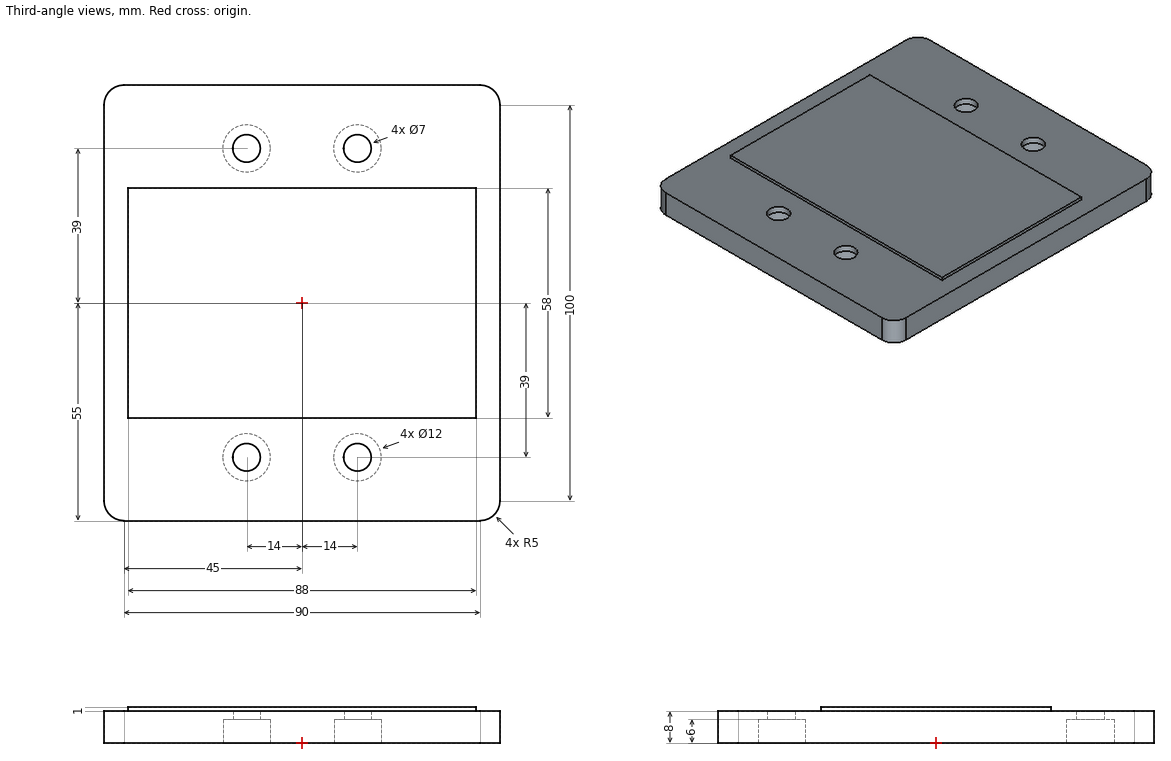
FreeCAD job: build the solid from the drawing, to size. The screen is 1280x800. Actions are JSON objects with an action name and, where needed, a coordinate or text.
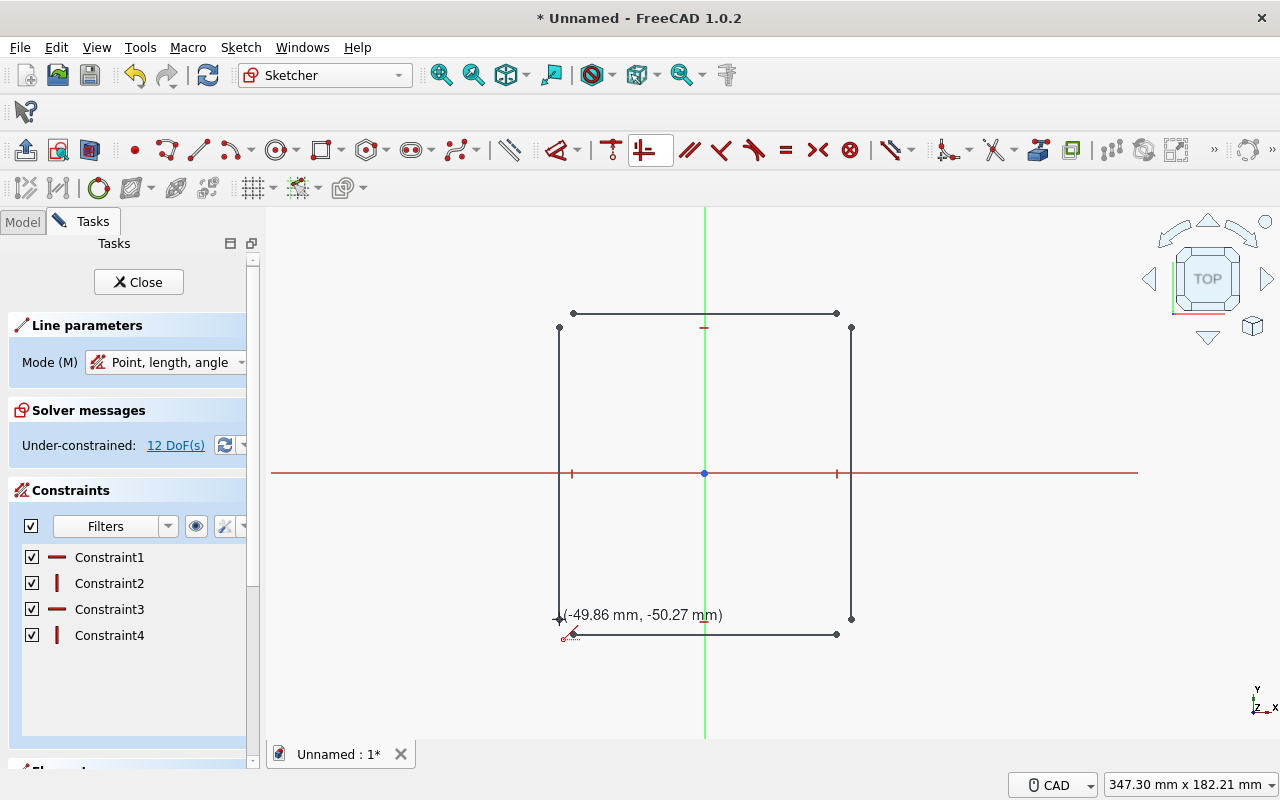
{"action": "left_click", "coordinate": [254, 150]}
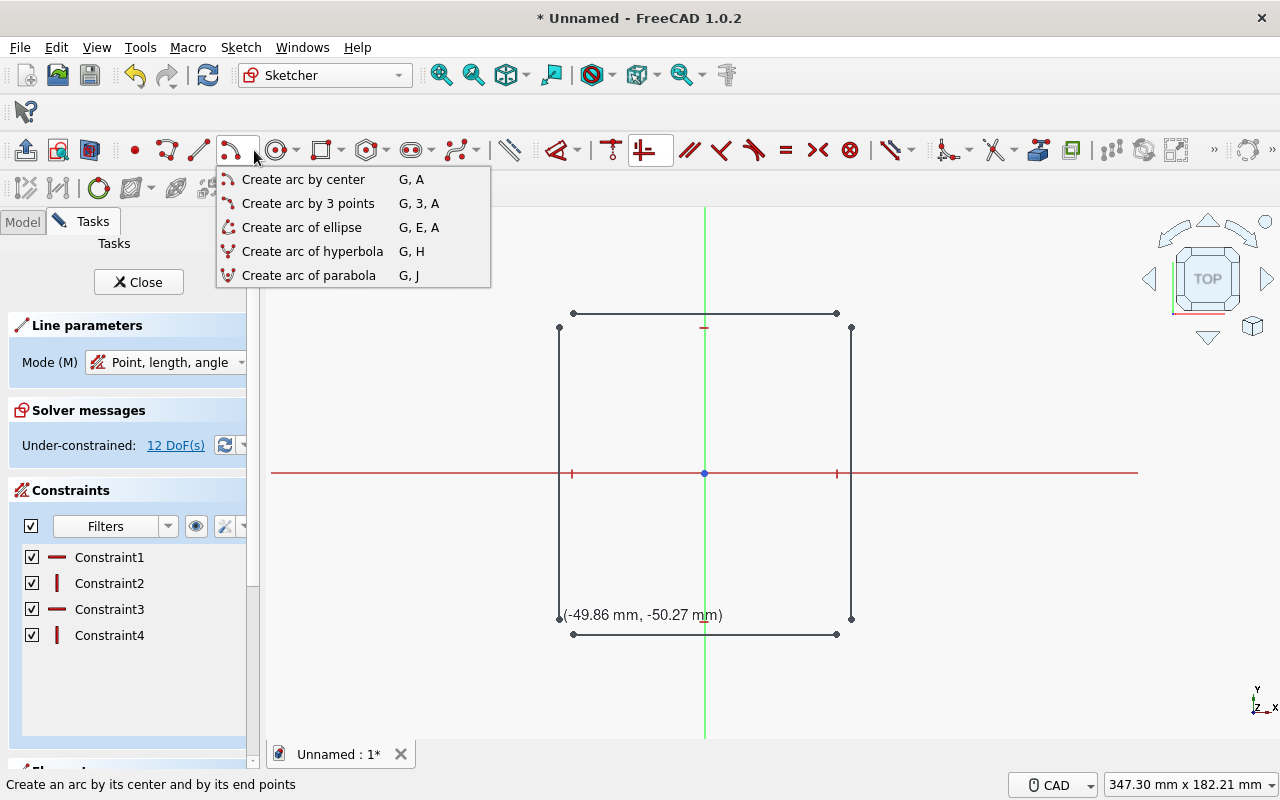
{"action": "left_click", "coordinate": [354, 203]}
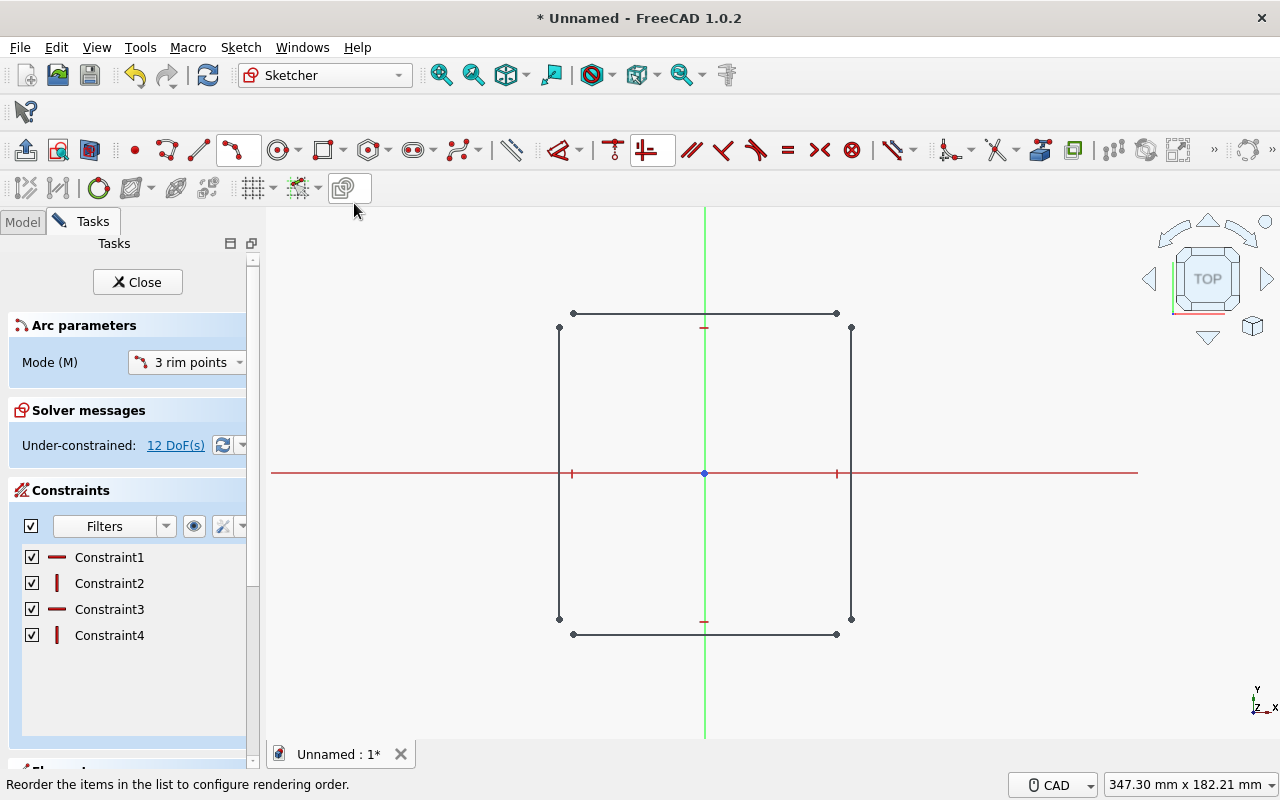
{"action": "left_click", "coordinate": [836, 635]}
{"action": "left_click", "coordinate": [851, 620]}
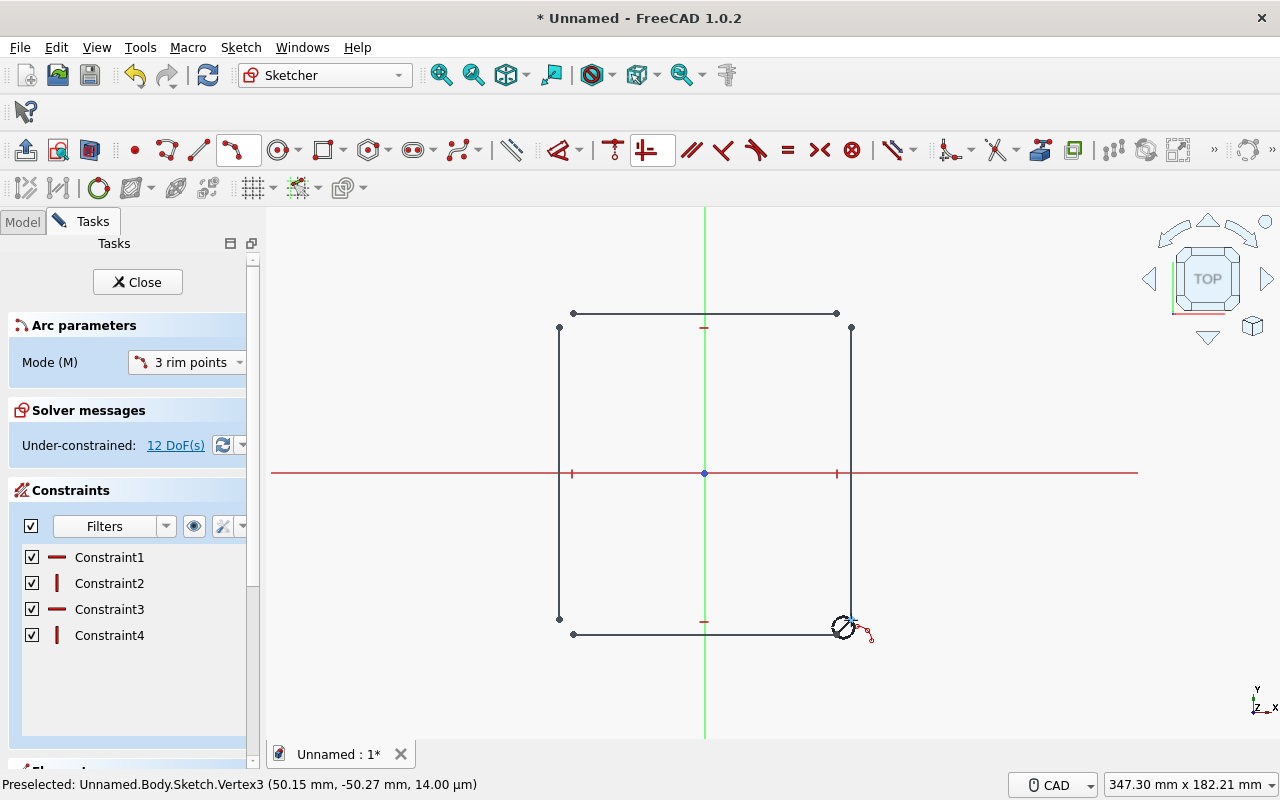
{"action": "scroll", "coordinate": [846, 630], "scroll_direction": "up", "scroll_amount": 7}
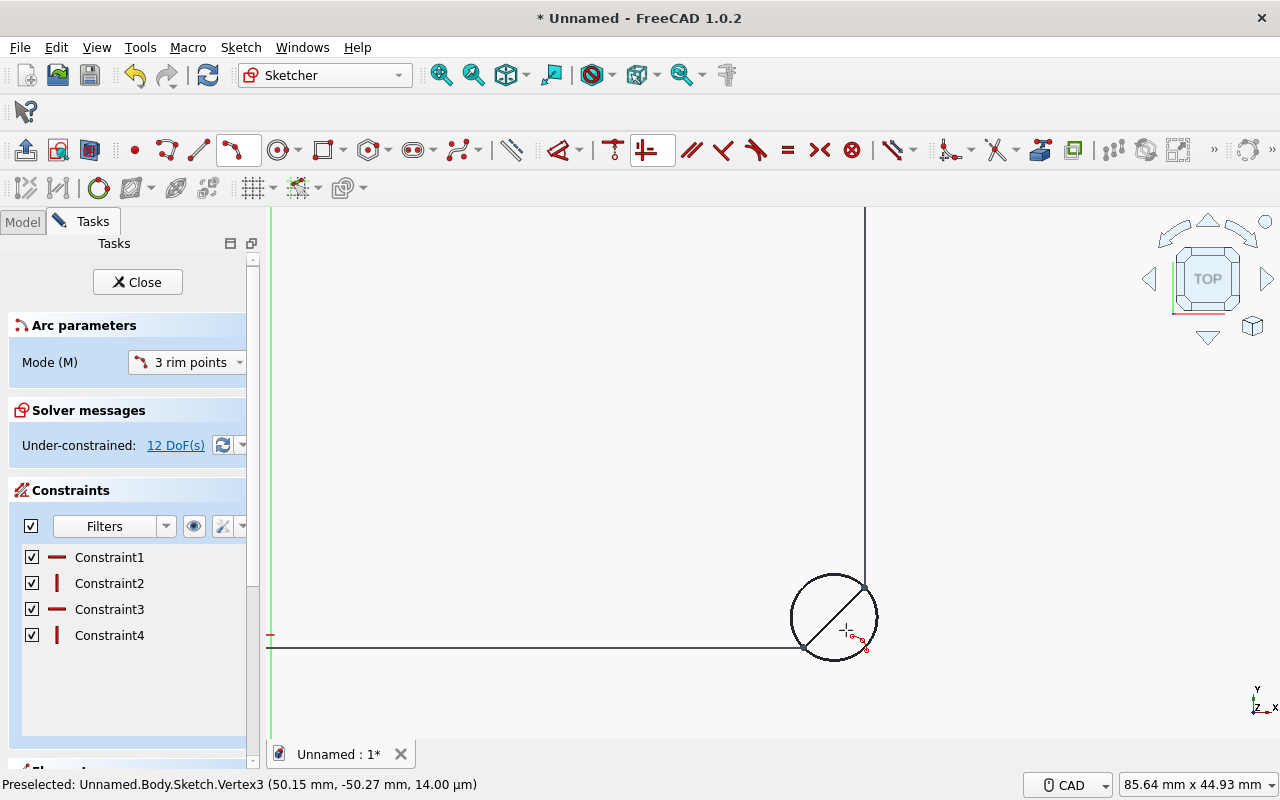
{"action": "left_click", "coordinate": [845, 626]}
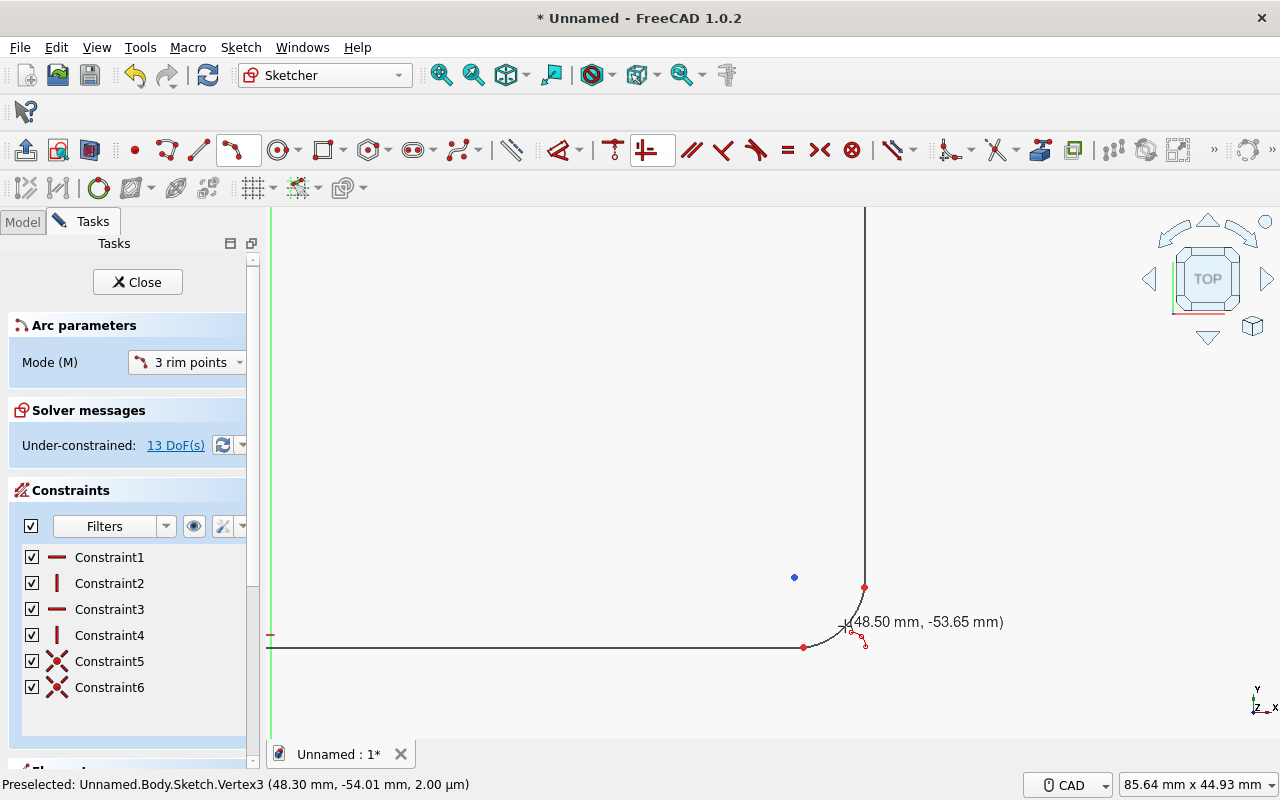
{"action": "scroll", "coordinate": [846, 630], "scroll_direction": "down", "scroll_amount": 7}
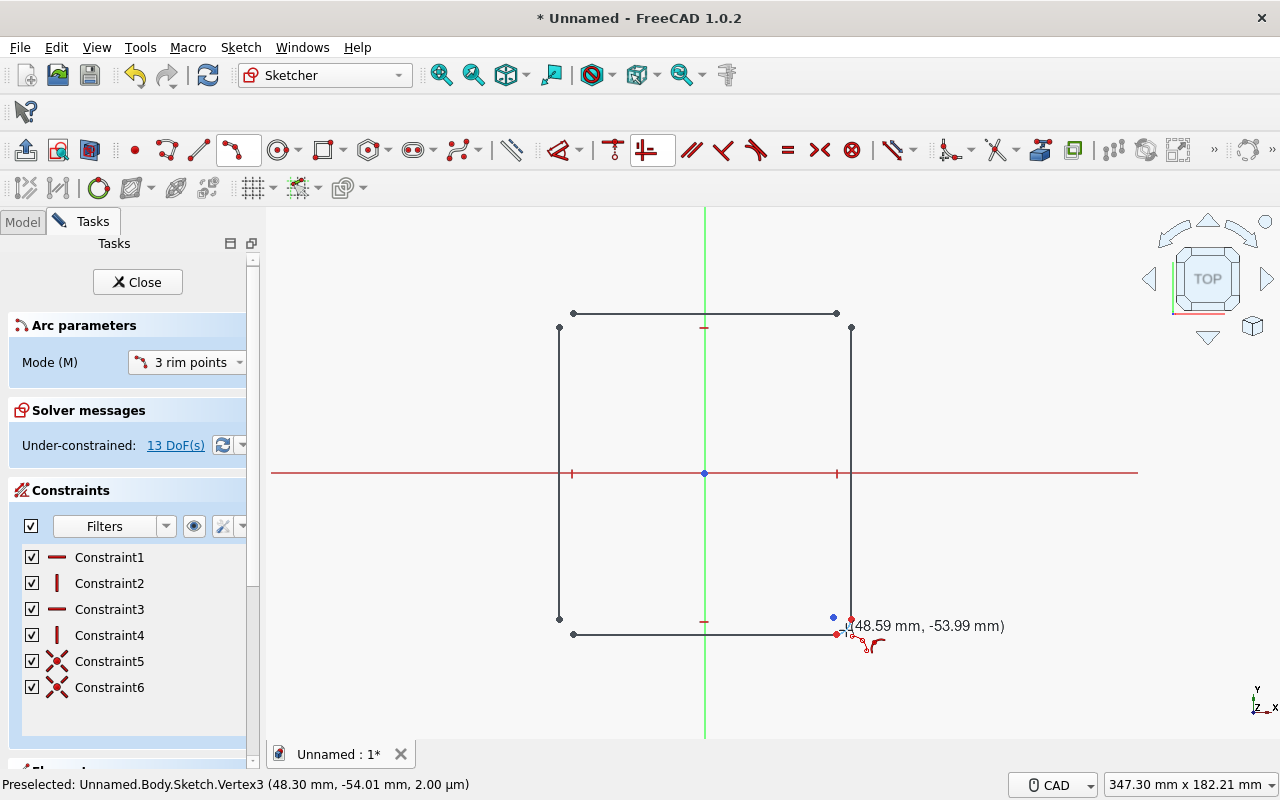
{"action": "left_click", "coordinate": [851, 328]}
{"action": "left_click", "coordinate": [836, 314]}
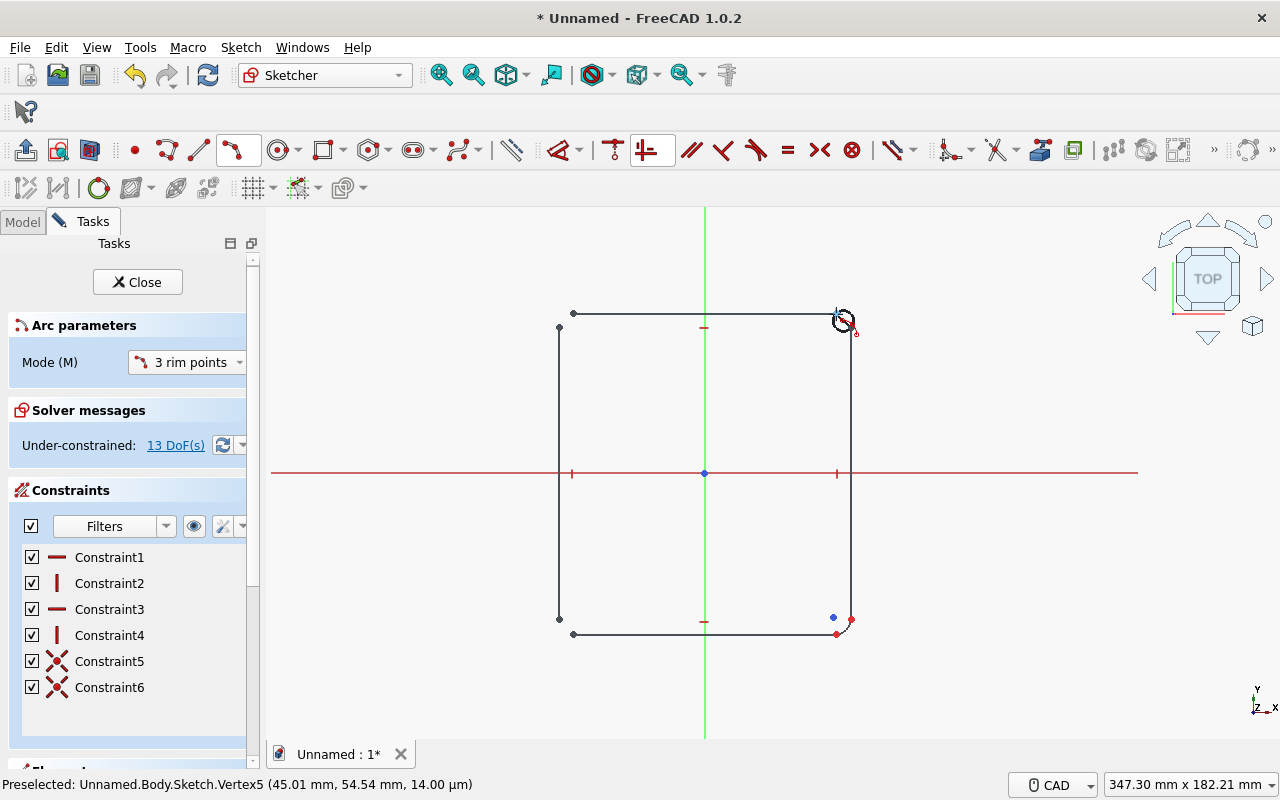
{"action": "scroll", "coordinate": [846, 317], "scroll_direction": "up", "scroll_amount": 7}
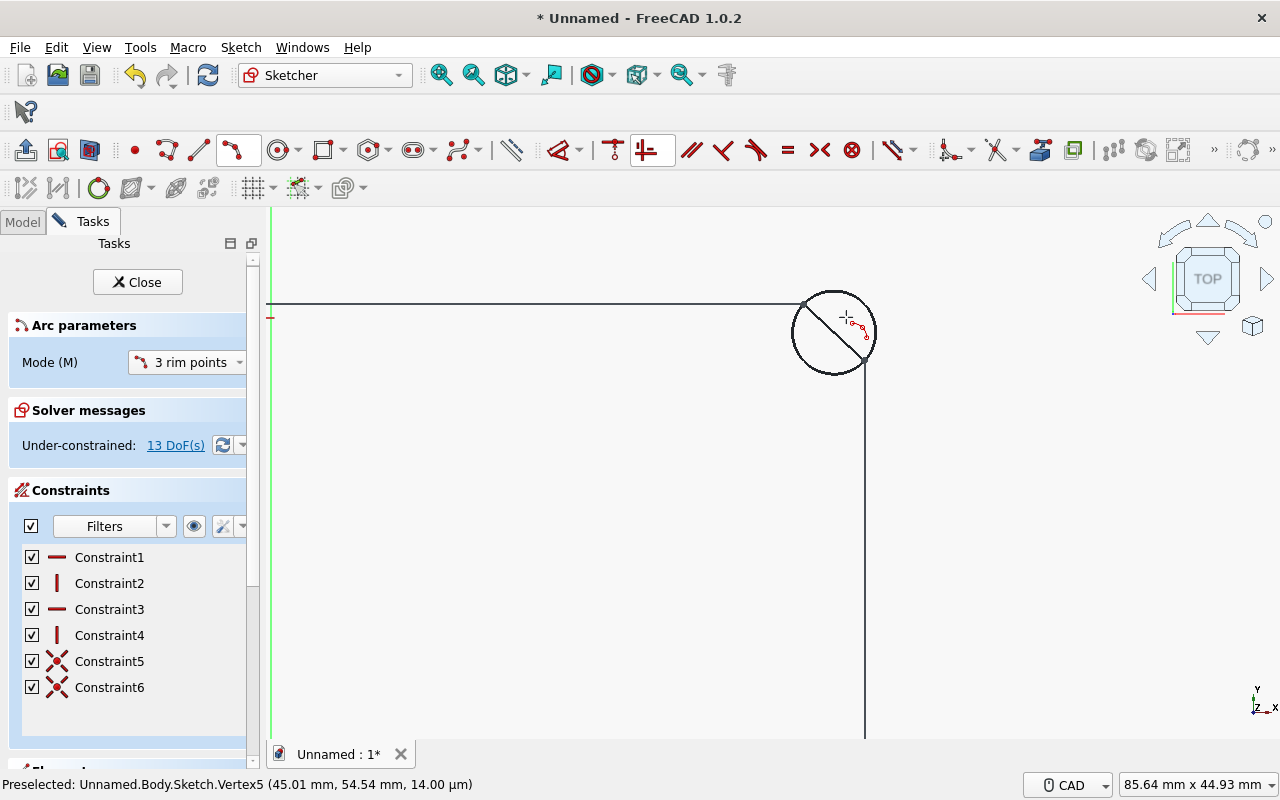
{"action": "left_click", "coordinate": [845, 316]}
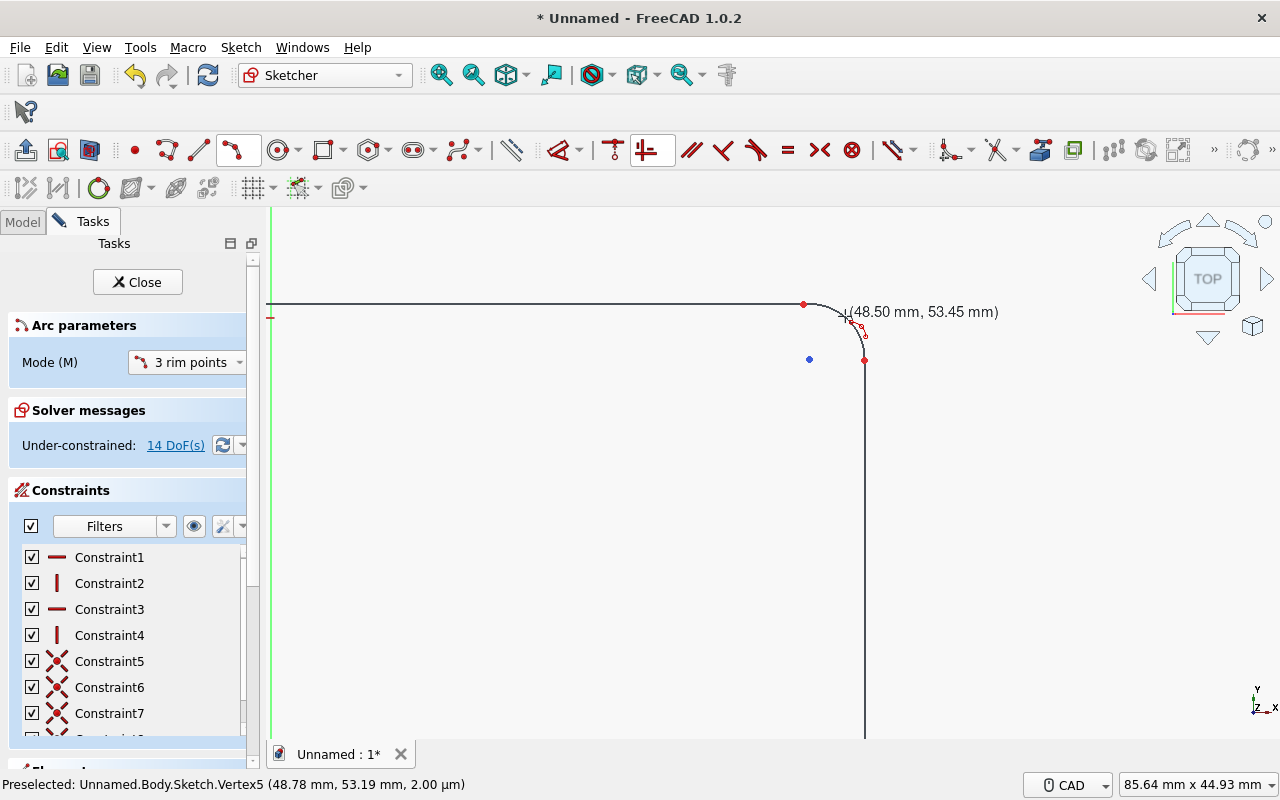
{"action": "scroll", "coordinate": [846, 317], "scroll_direction": "down", "scroll_amount": 7}